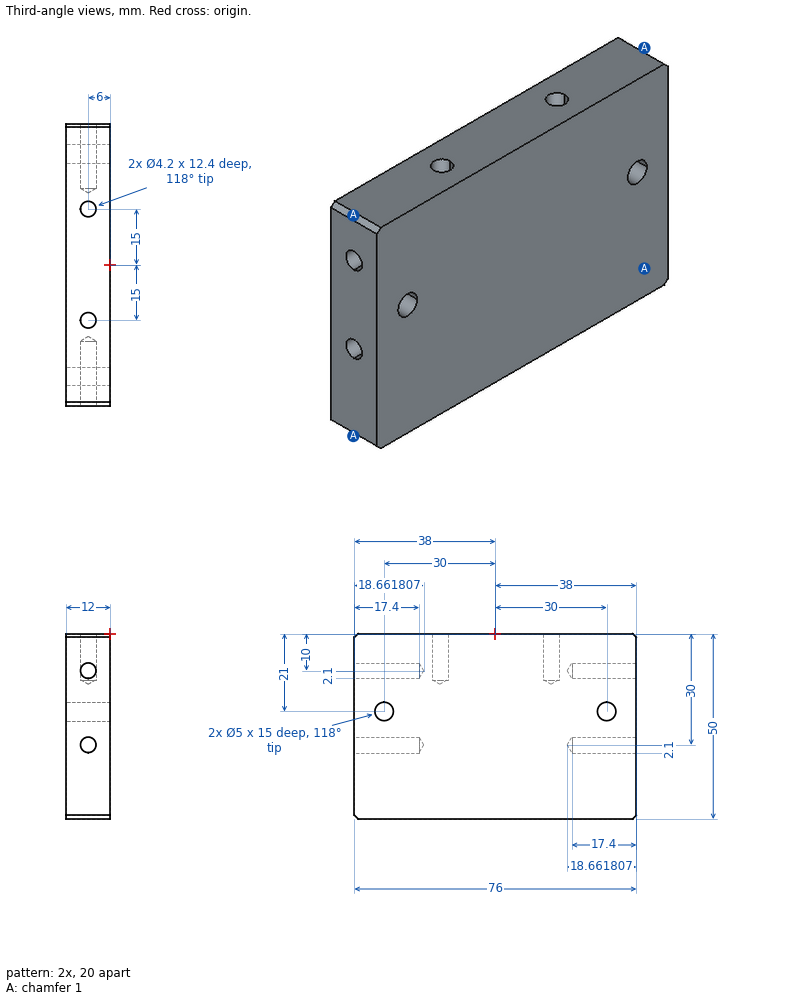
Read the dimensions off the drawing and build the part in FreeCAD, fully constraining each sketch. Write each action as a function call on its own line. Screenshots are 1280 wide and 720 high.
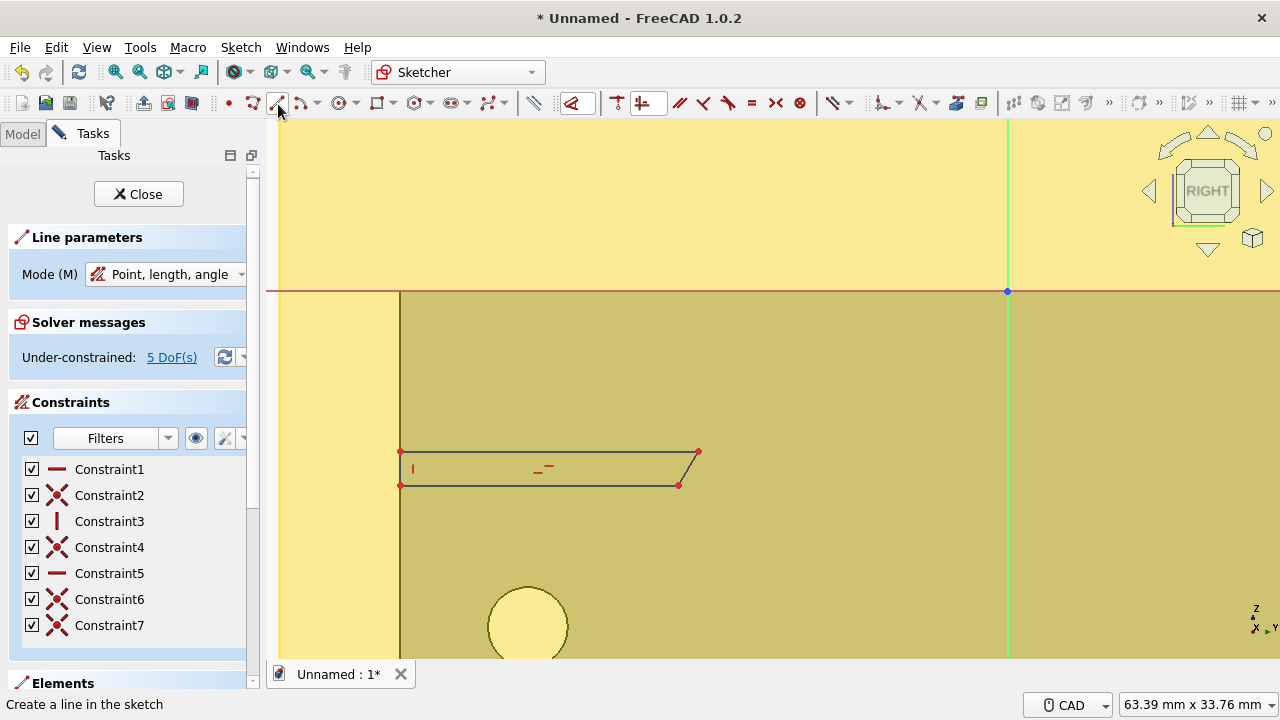
click(728, 451)
click(818, 451)
key(Escape)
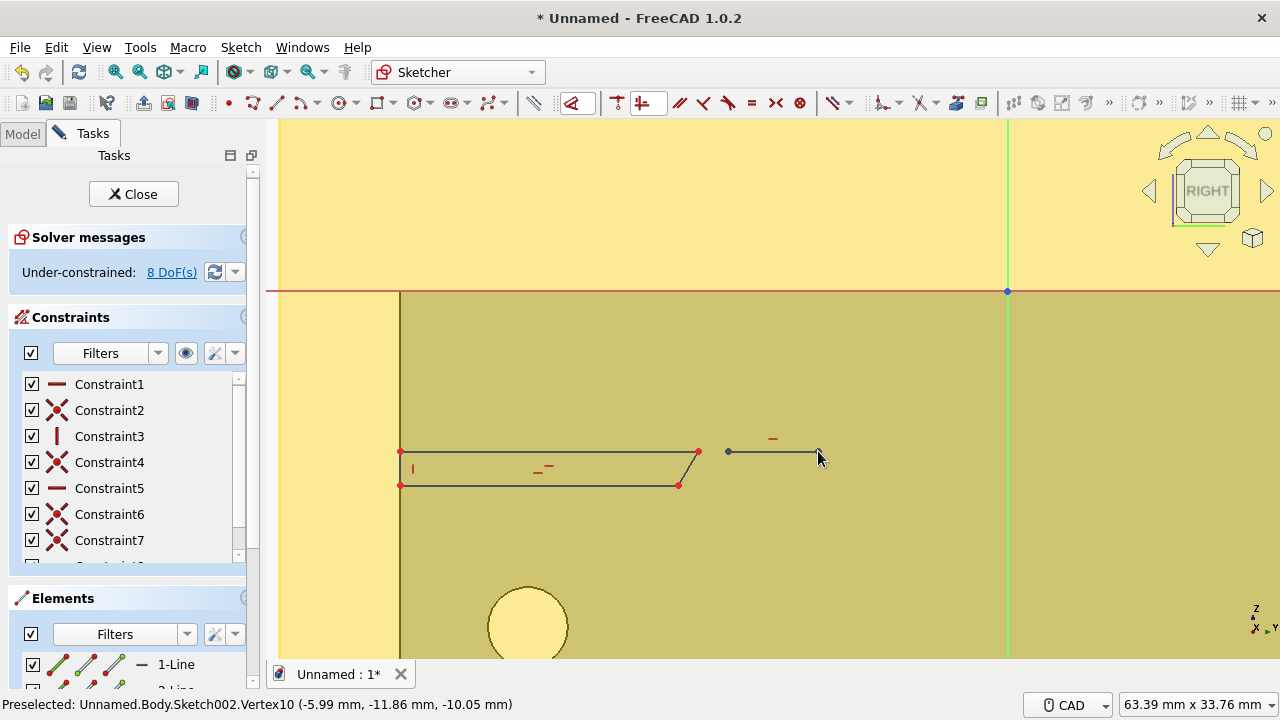
click(755, 452)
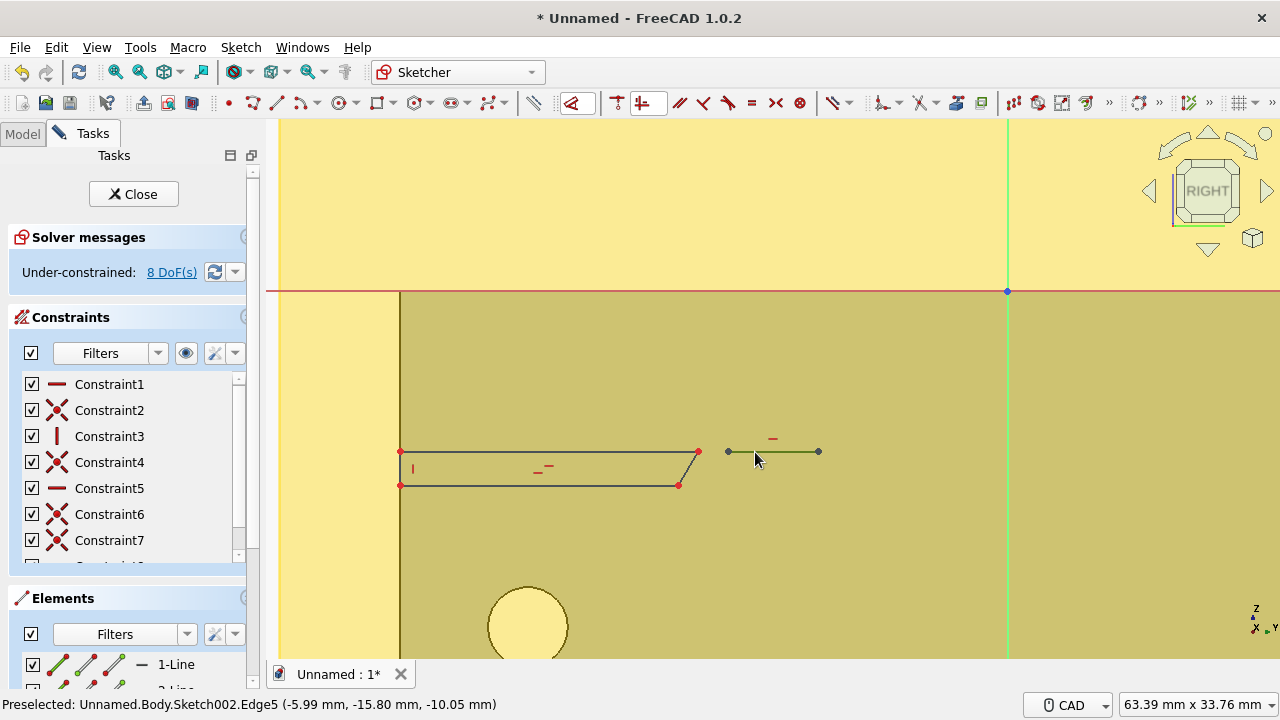
key(g)
key(n)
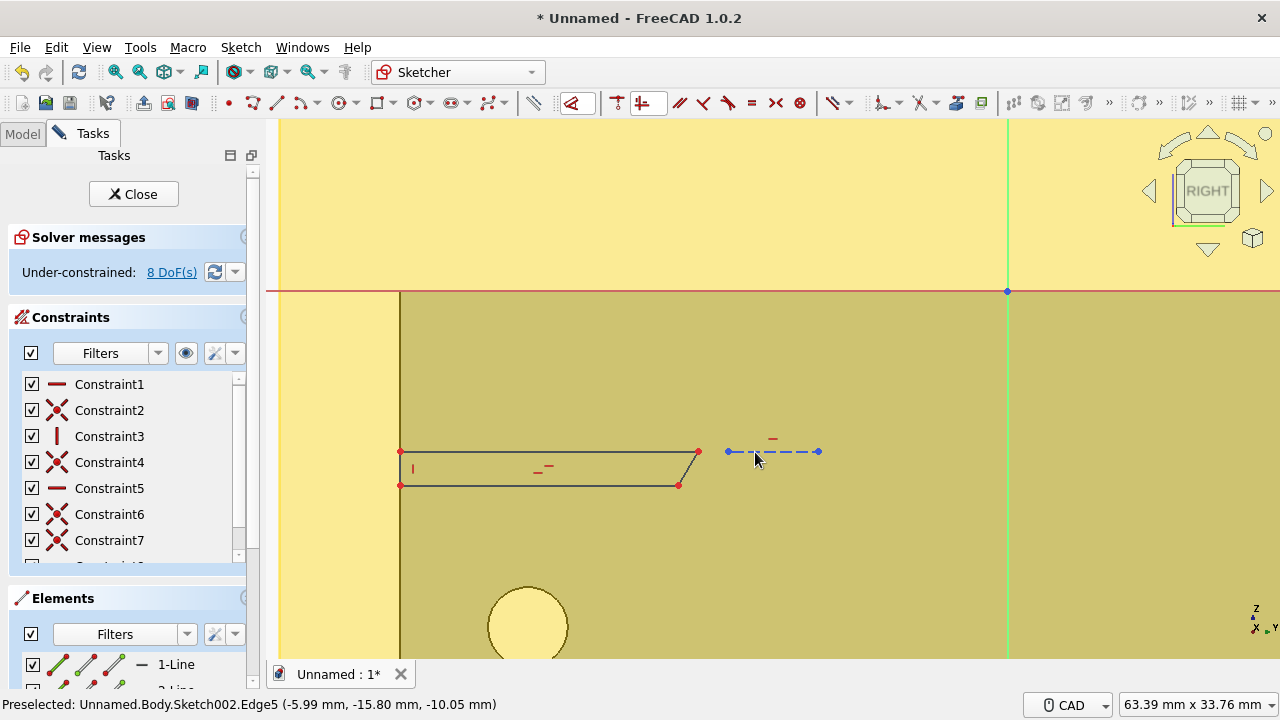
scroll(400, 462, up, 2)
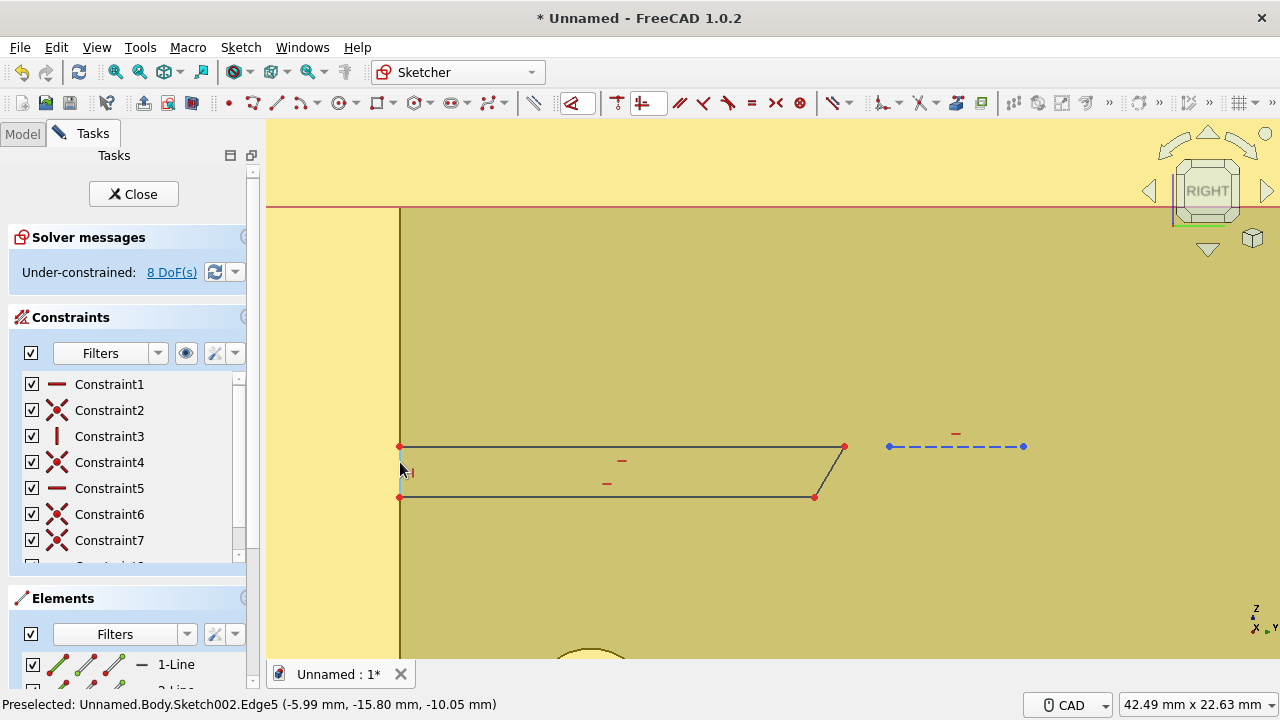
click(400, 462)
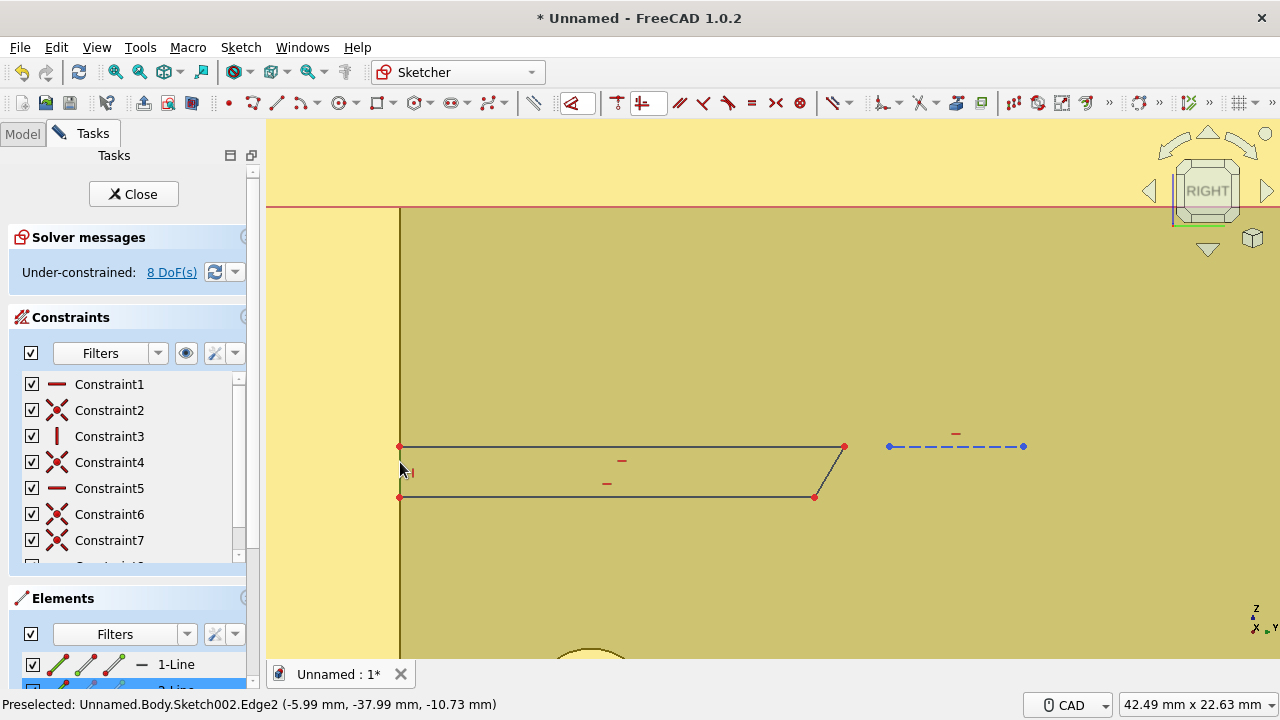
click(590, 104)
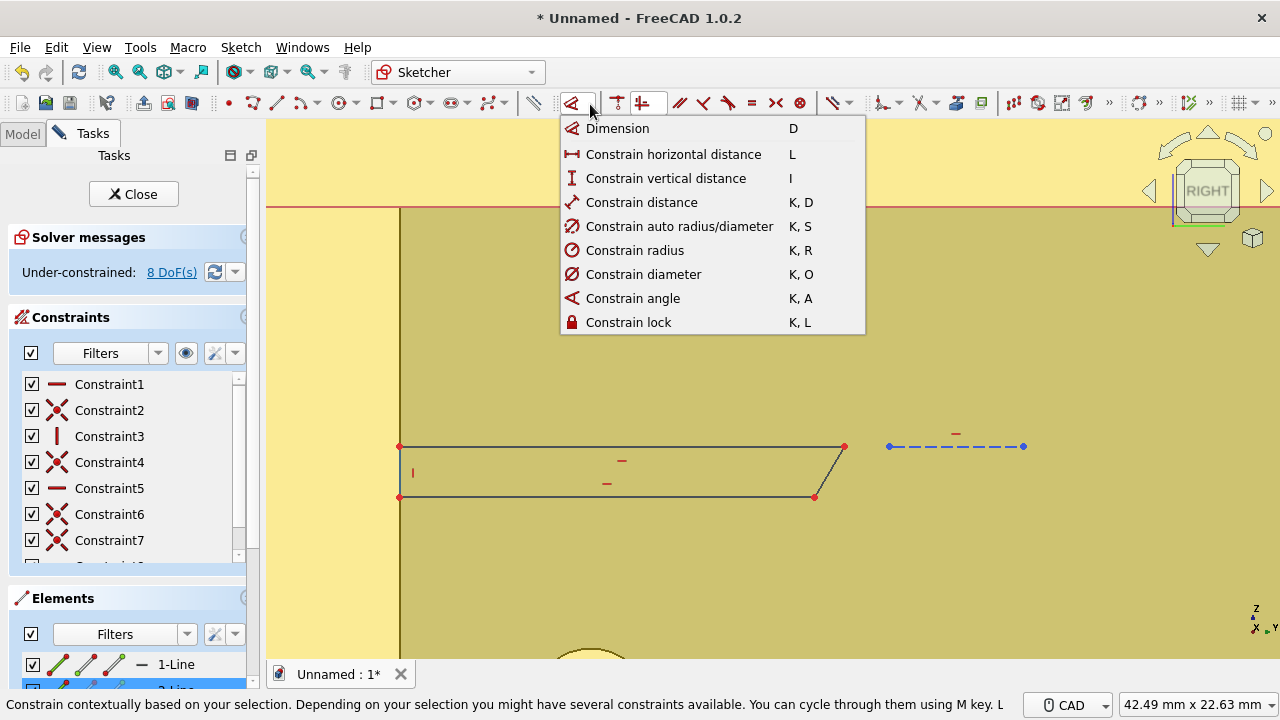
click(713, 178)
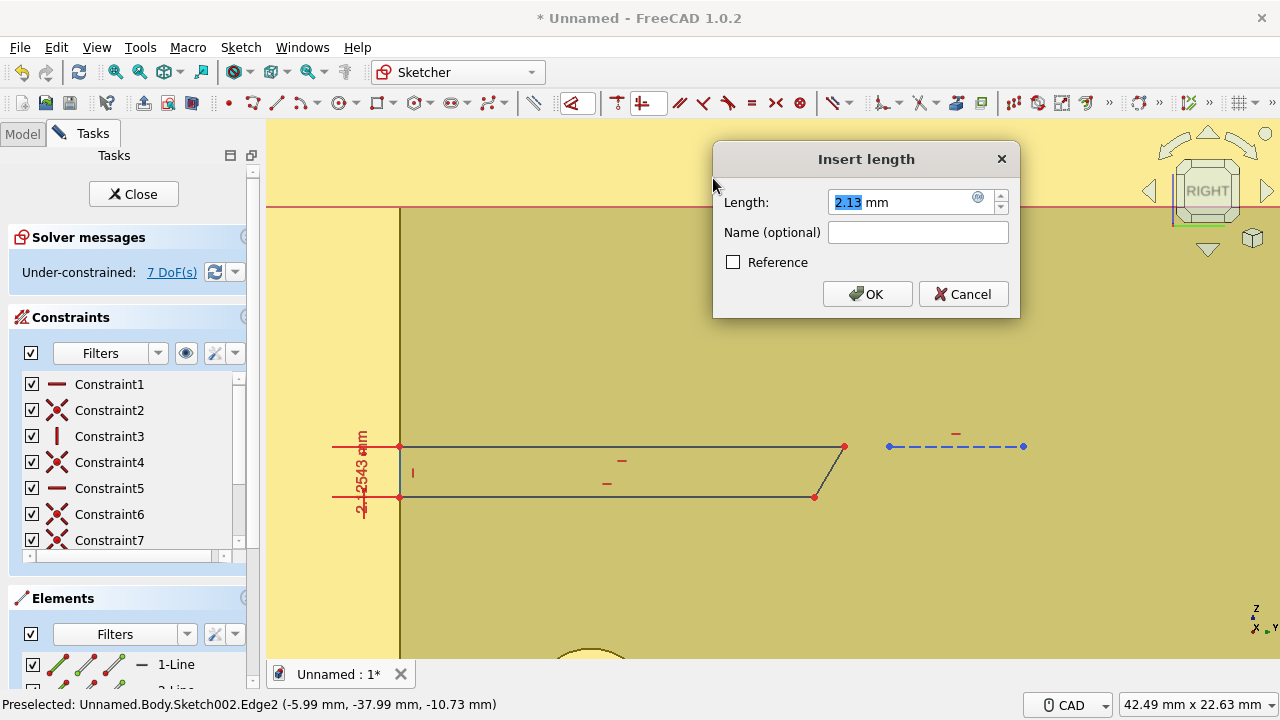
text(2.1)
key(Return)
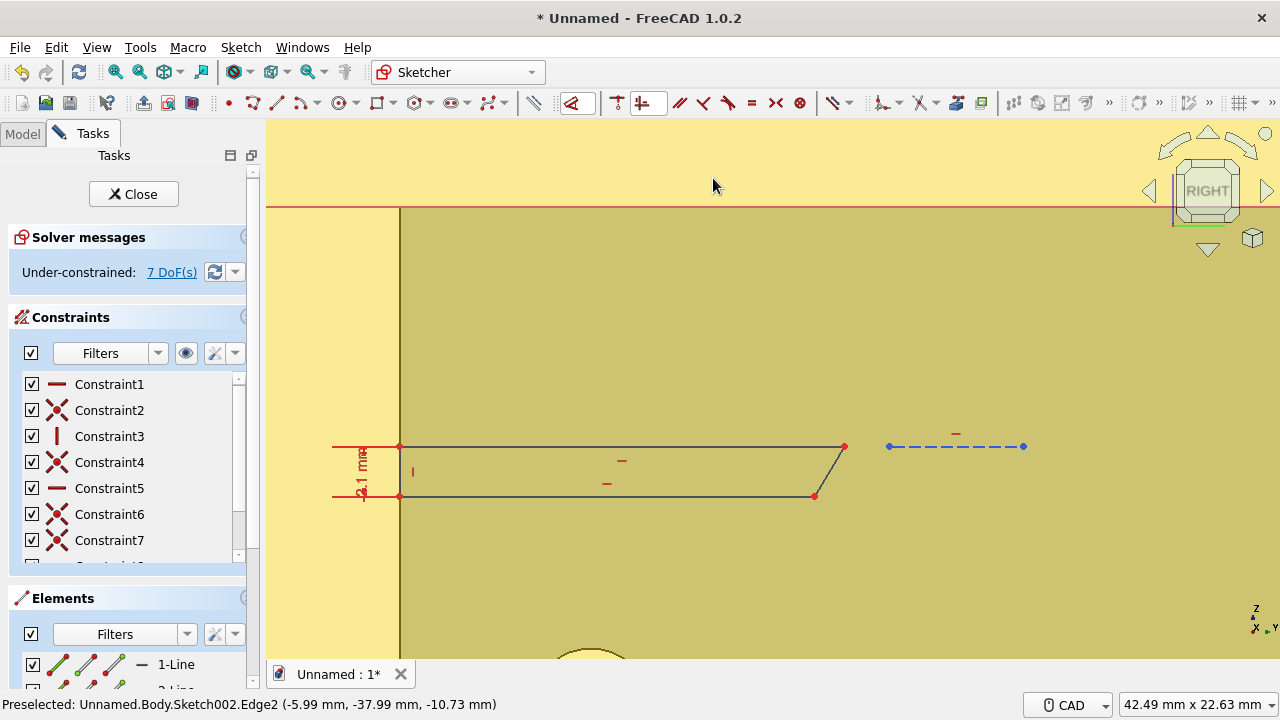
click(844, 447)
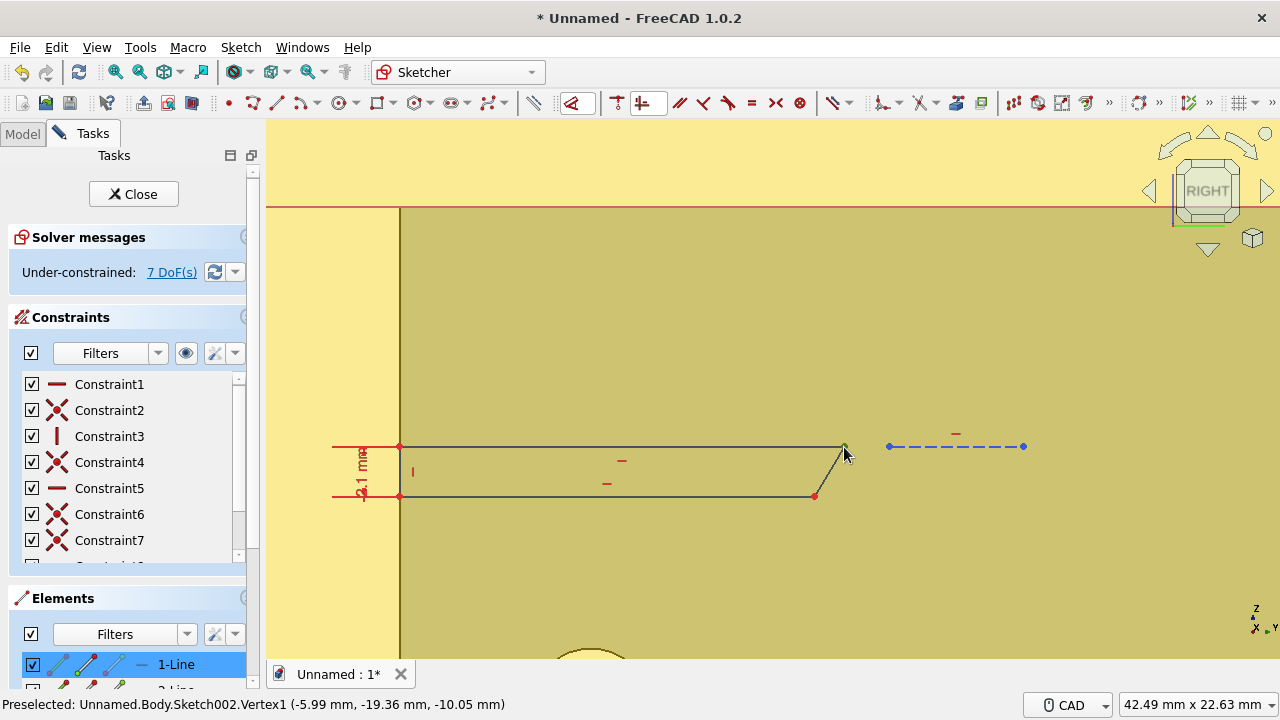
key(i)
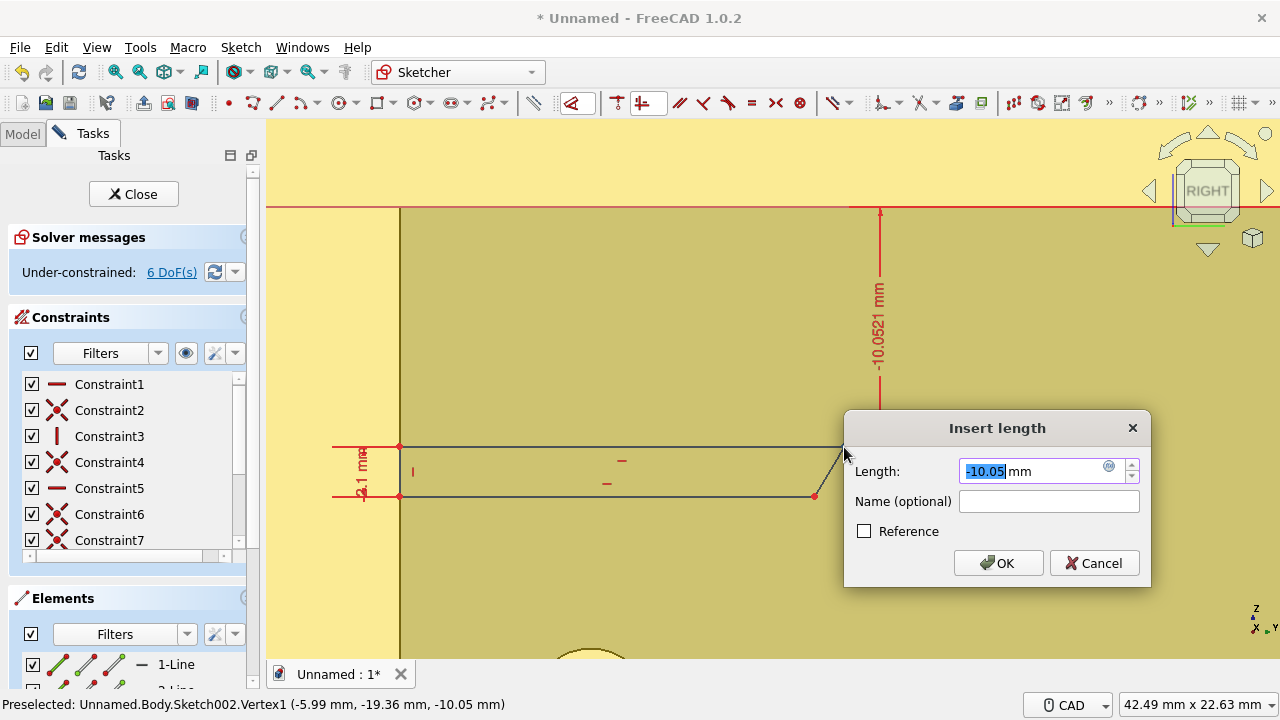
text(-10)
key(Return)